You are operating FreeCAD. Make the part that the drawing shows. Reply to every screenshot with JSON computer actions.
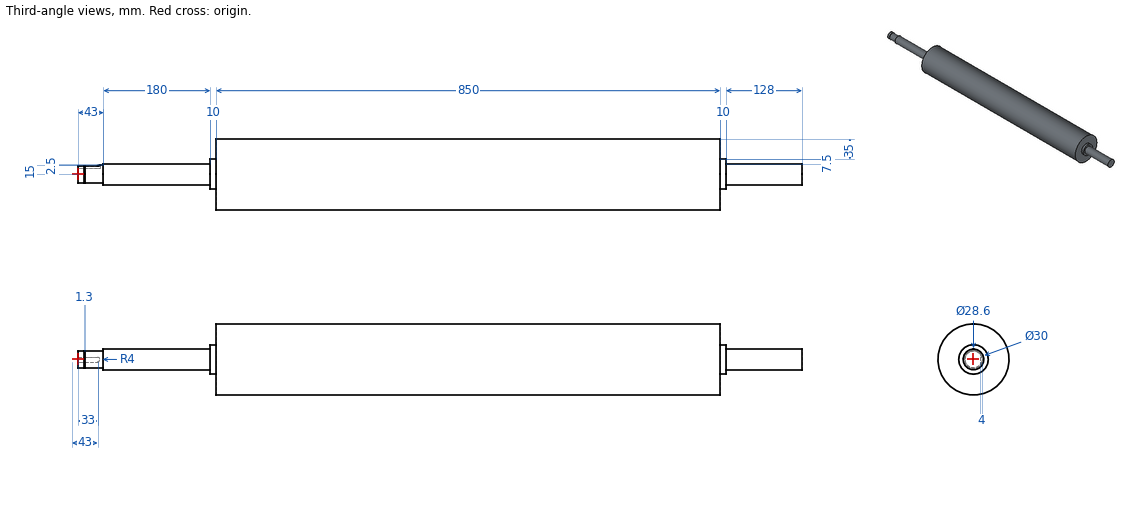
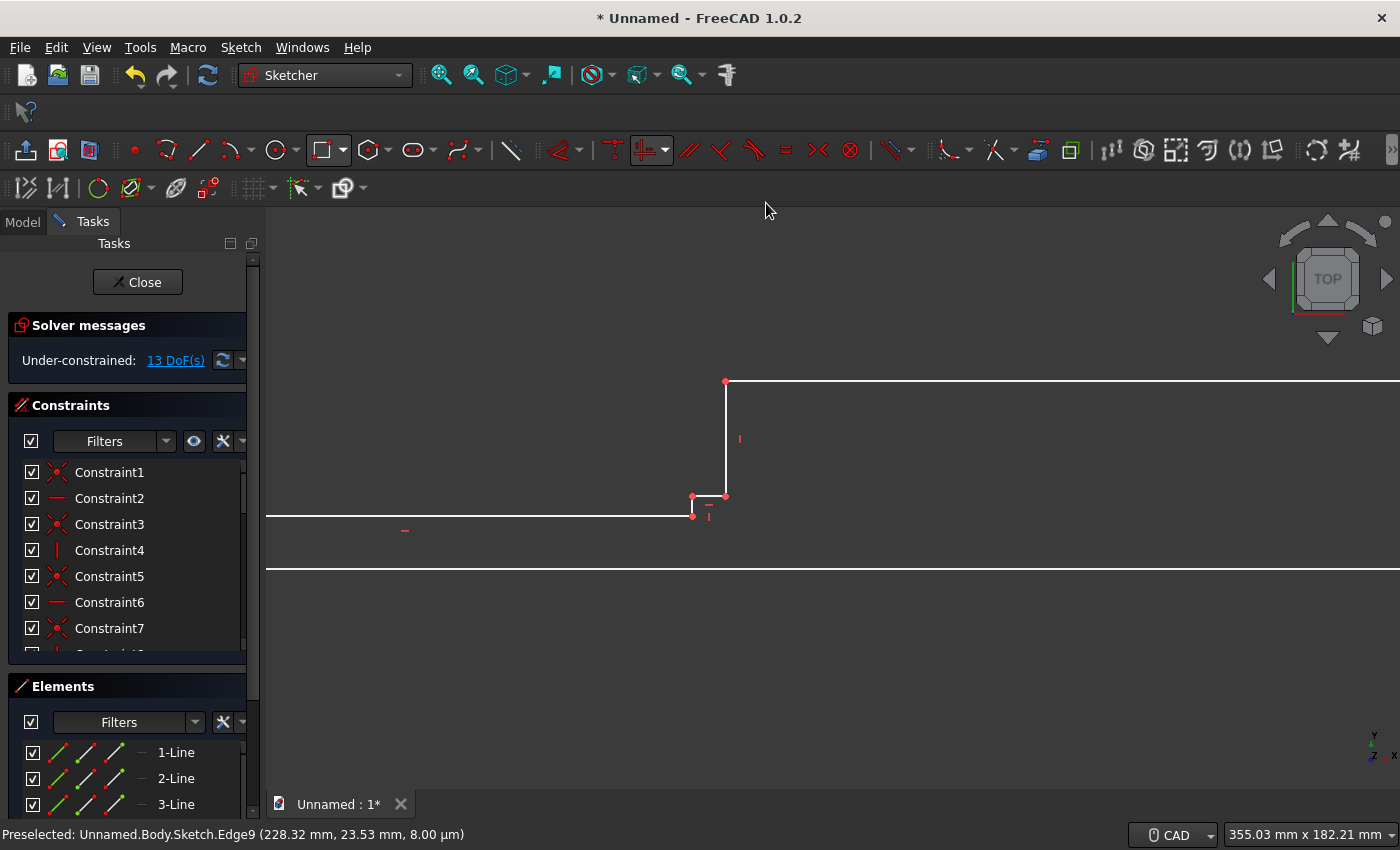
{"action": "scroll", "coordinate": [534, 503], "scroll_direction": "down", "scroll_amount": 9}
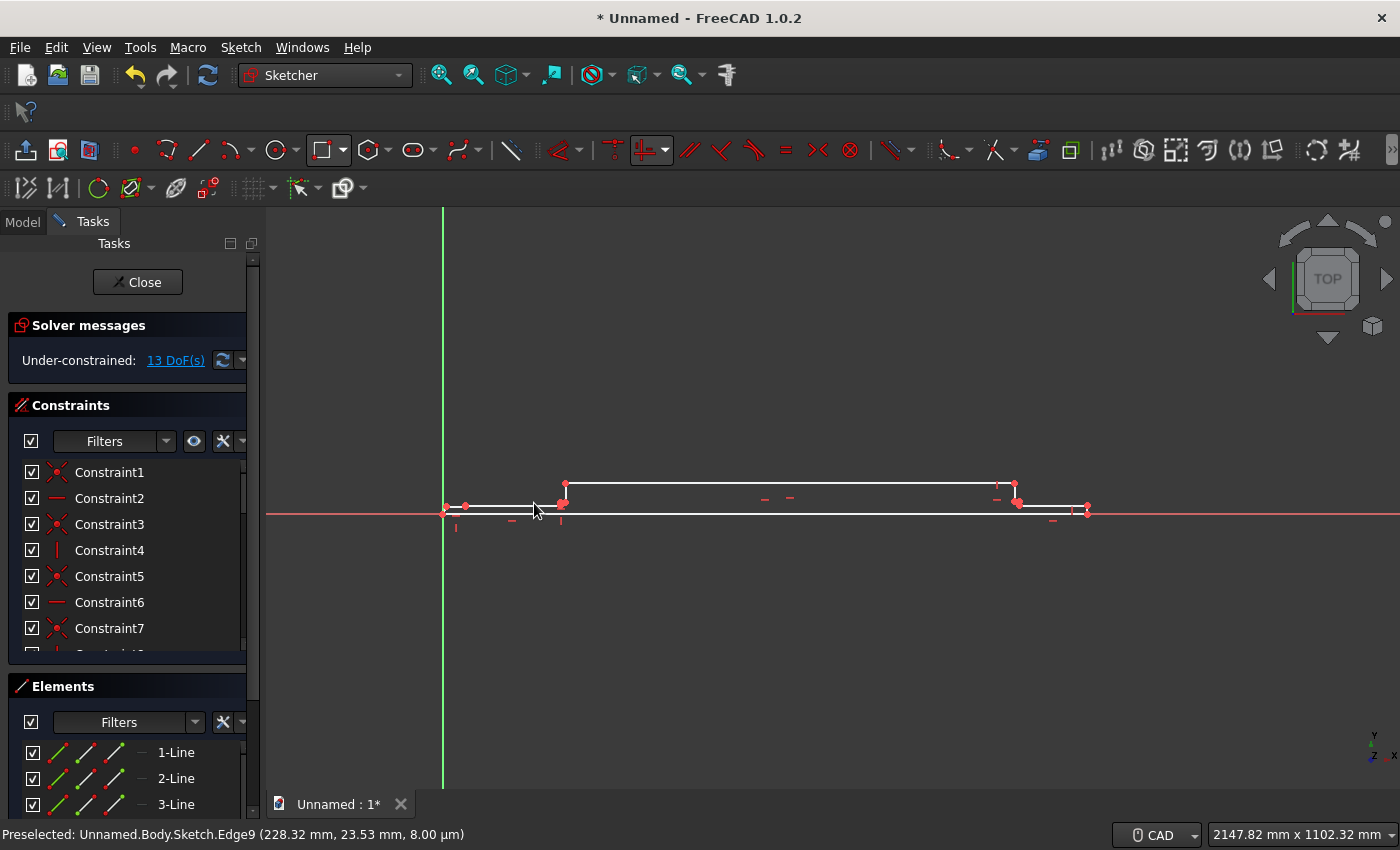
{"action": "scroll", "coordinate": [445, 509], "scroll_direction": "up", "scroll_amount": 9}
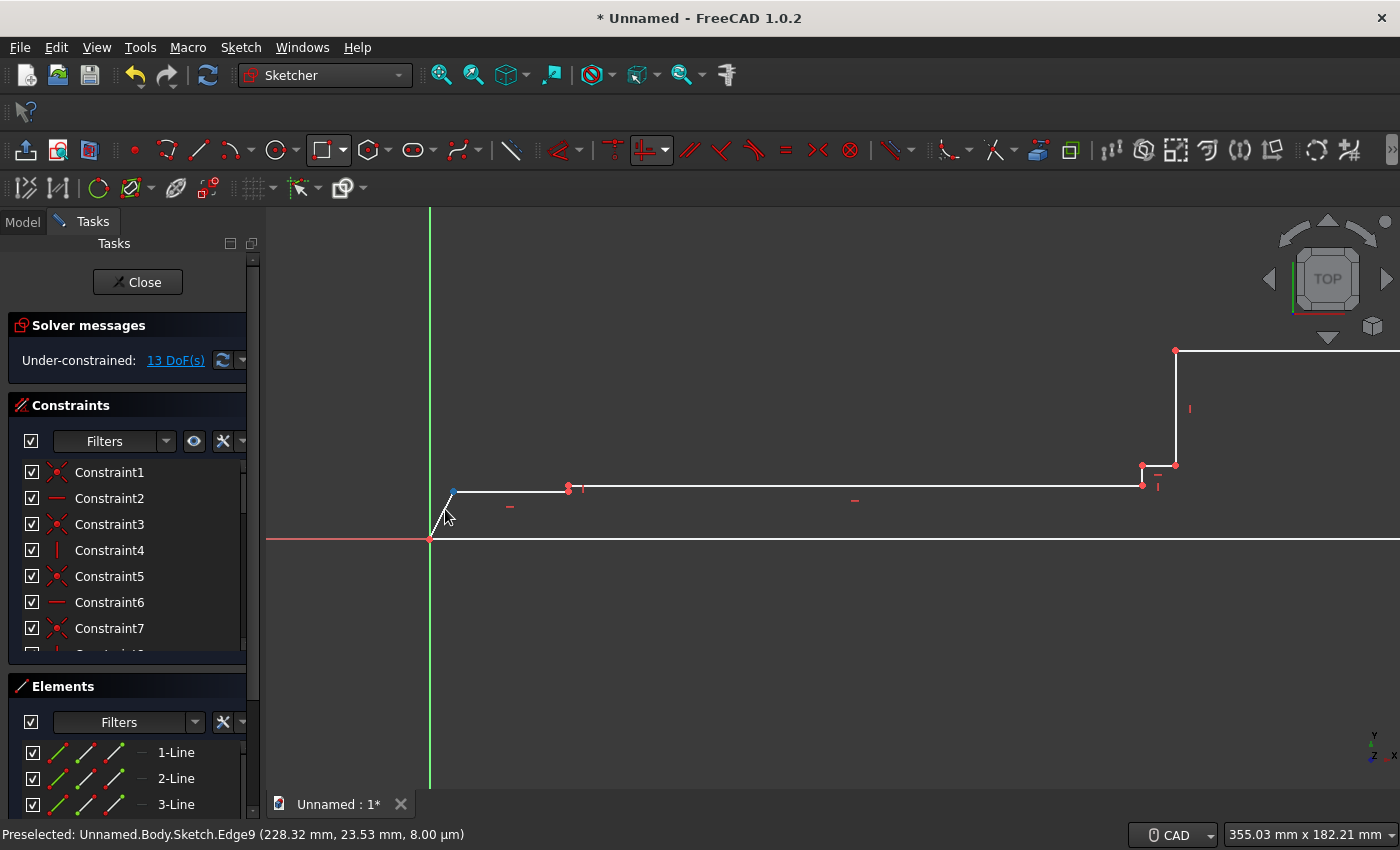
{"action": "left_click", "coordinate": [446, 506]}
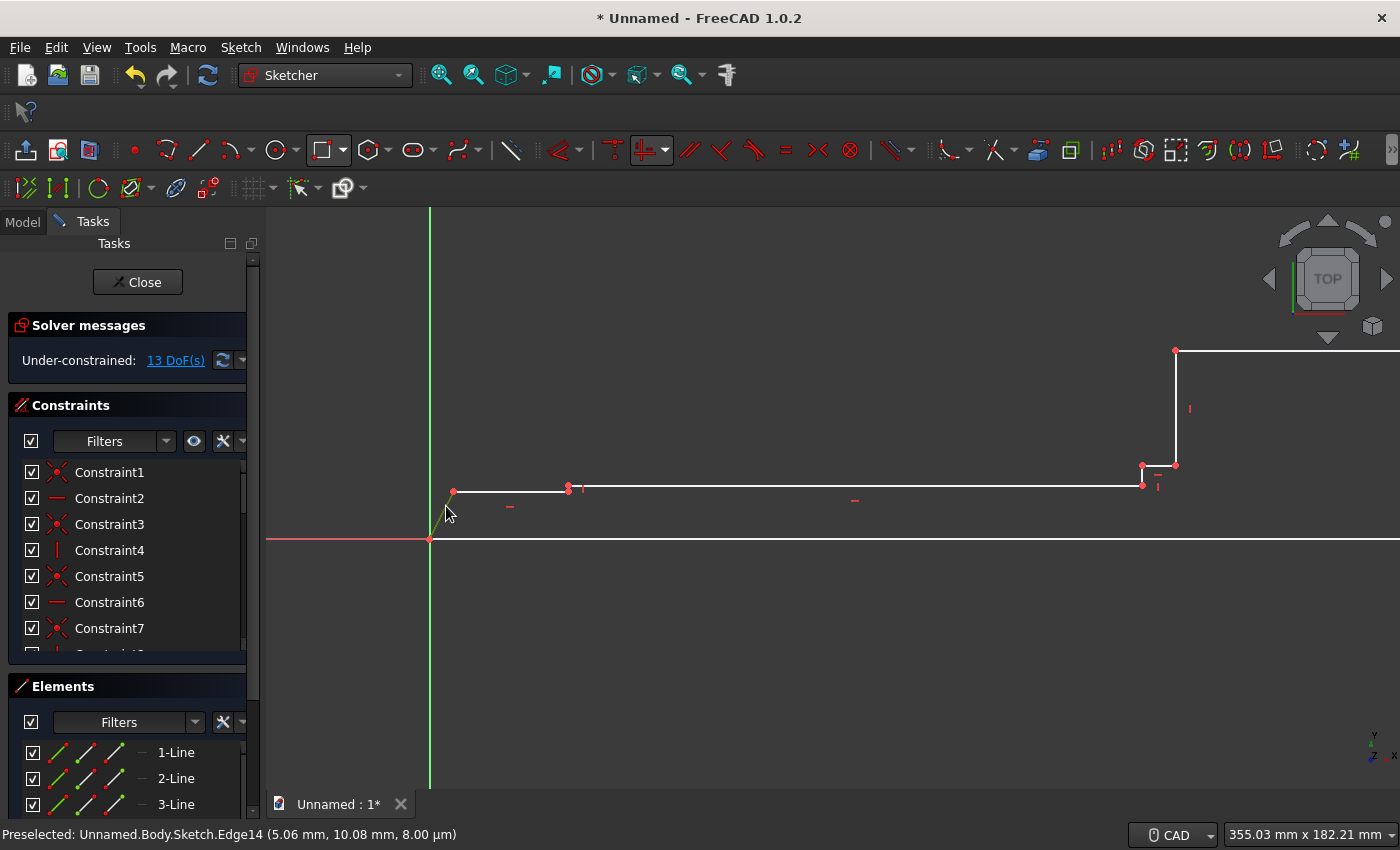
{"action": "left_click", "coordinate": [668, 150]}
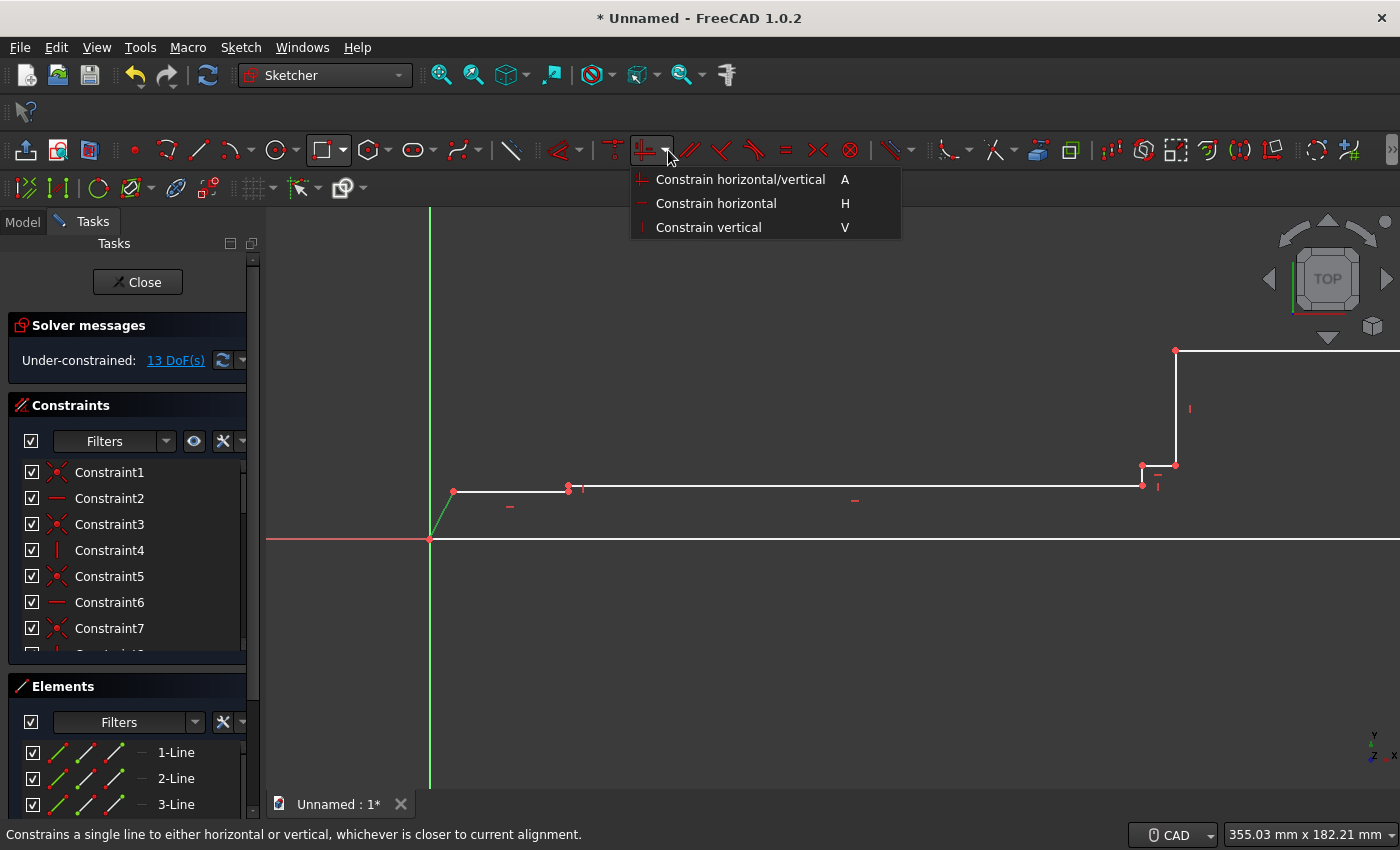
{"action": "left_click", "coordinate": [766, 227]}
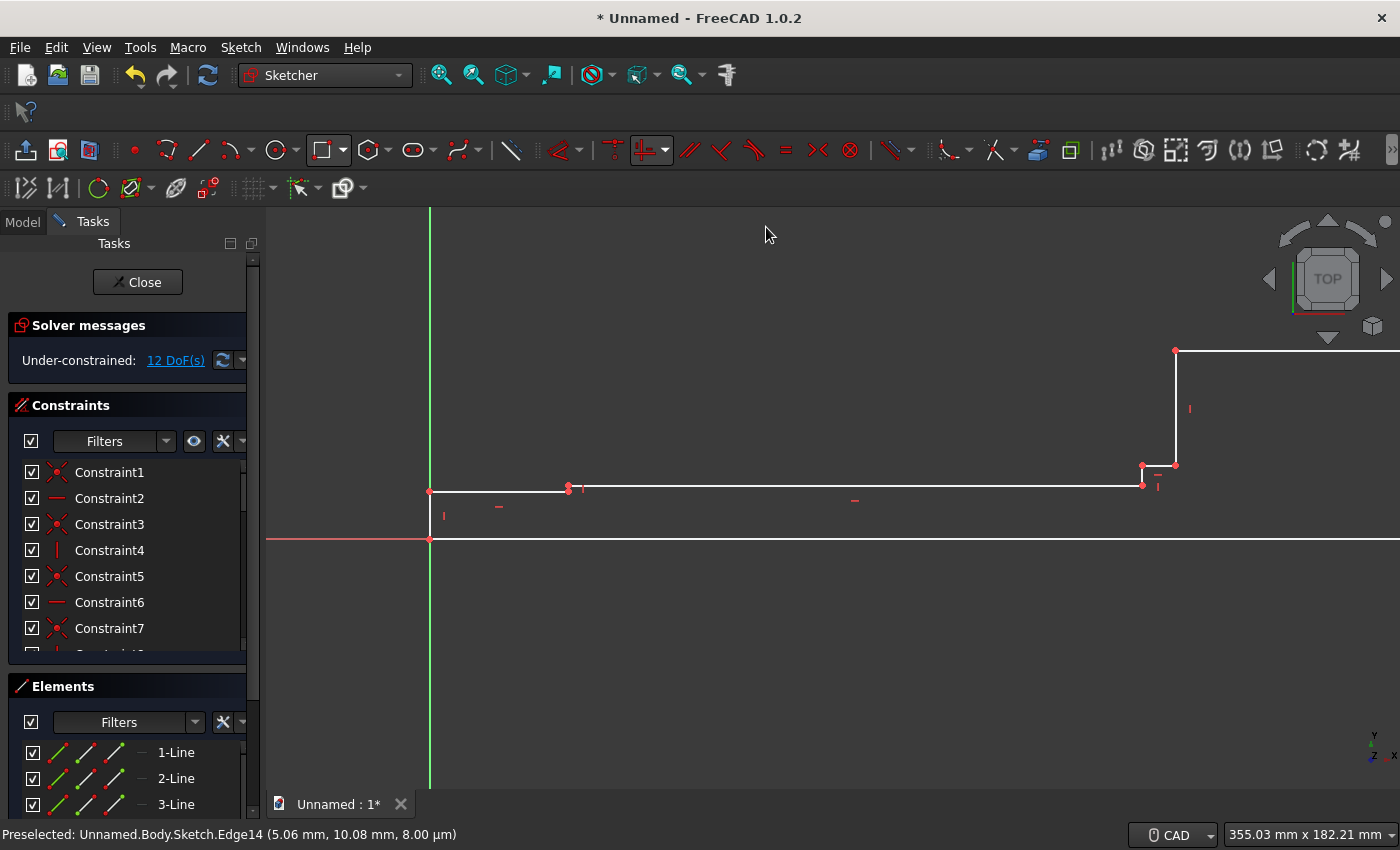
{"action": "left_click", "coordinate": [558, 150]}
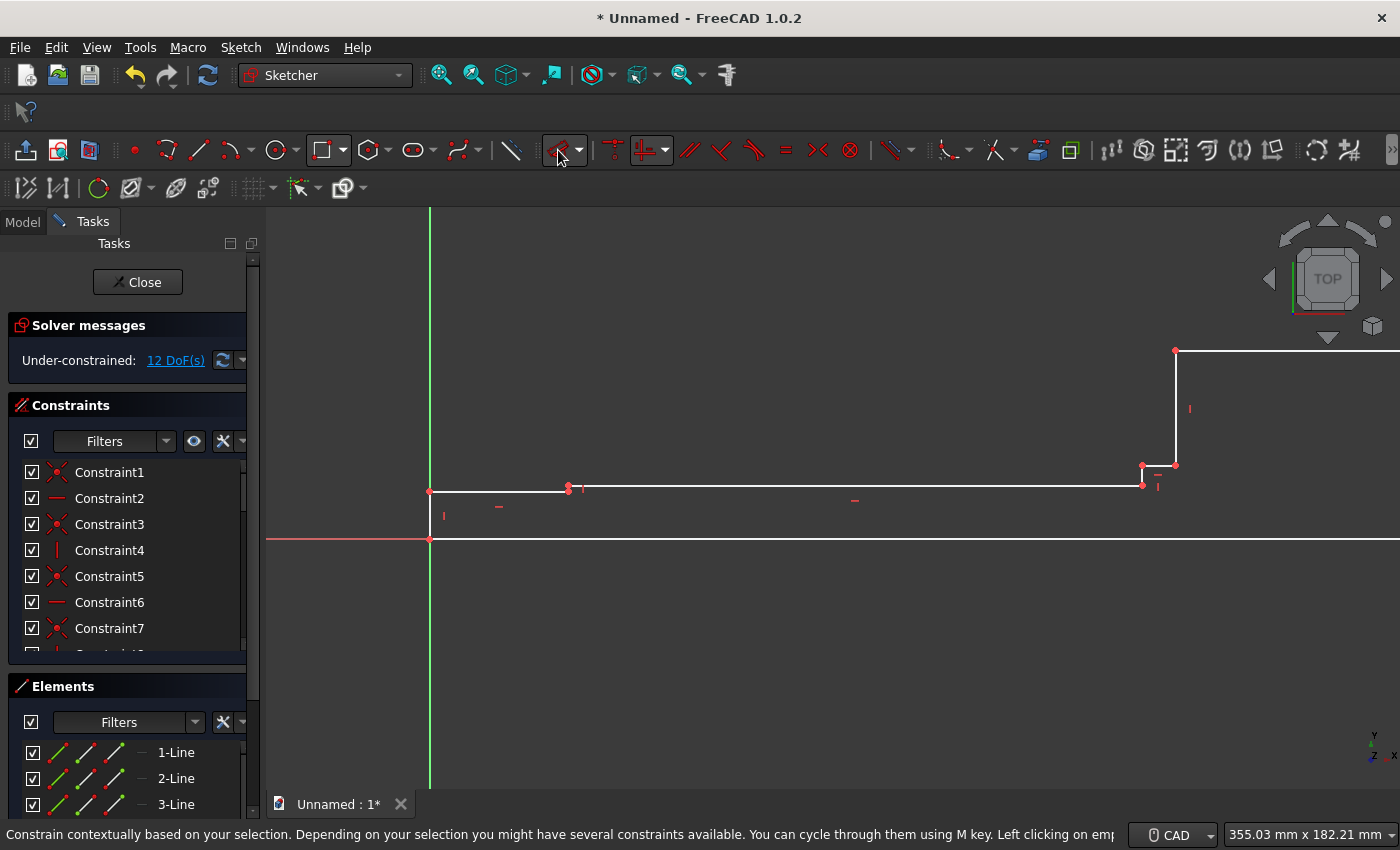
{"action": "scroll", "coordinate": [445, 509], "scroll_direction": "down", "scroll_amount": 9}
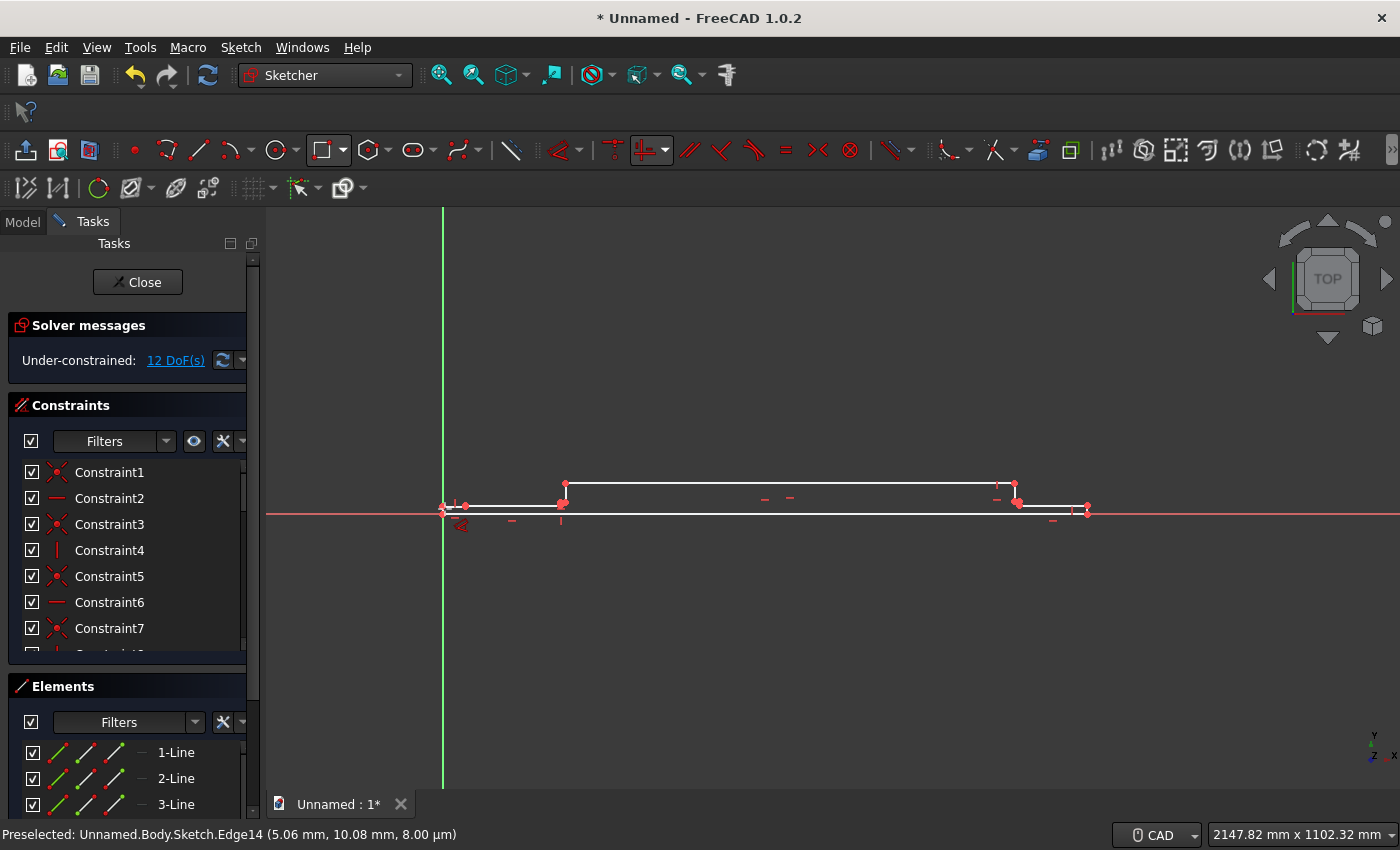
{"action": "scroll", "coordinate": [1018, 501], "scroll_direction": "up", "scroll_amount": 11}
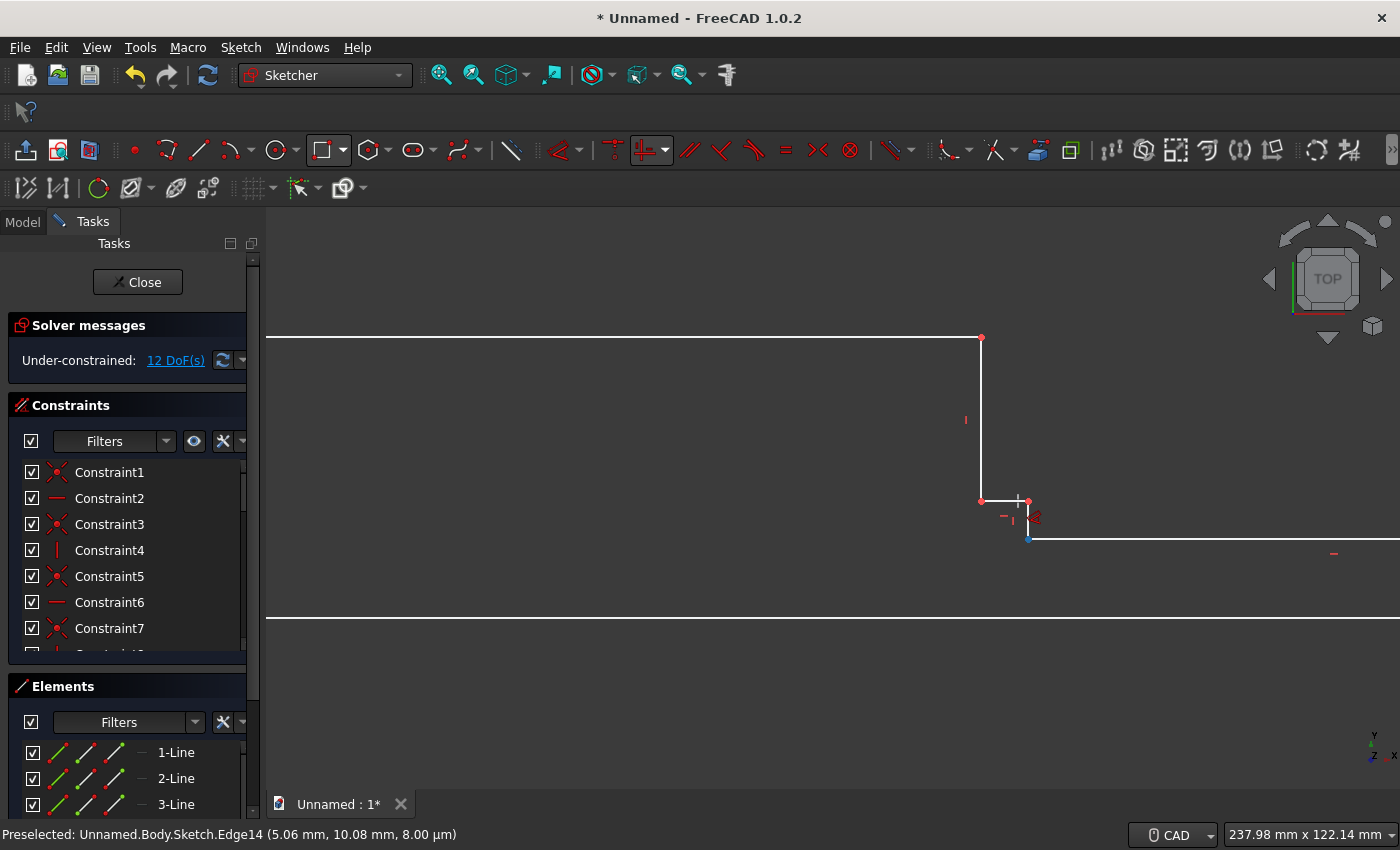
{"action": "left_click", "coordinate": [1014, 501]}
{"action": "left_click", "coordinate": [1005, 535]}